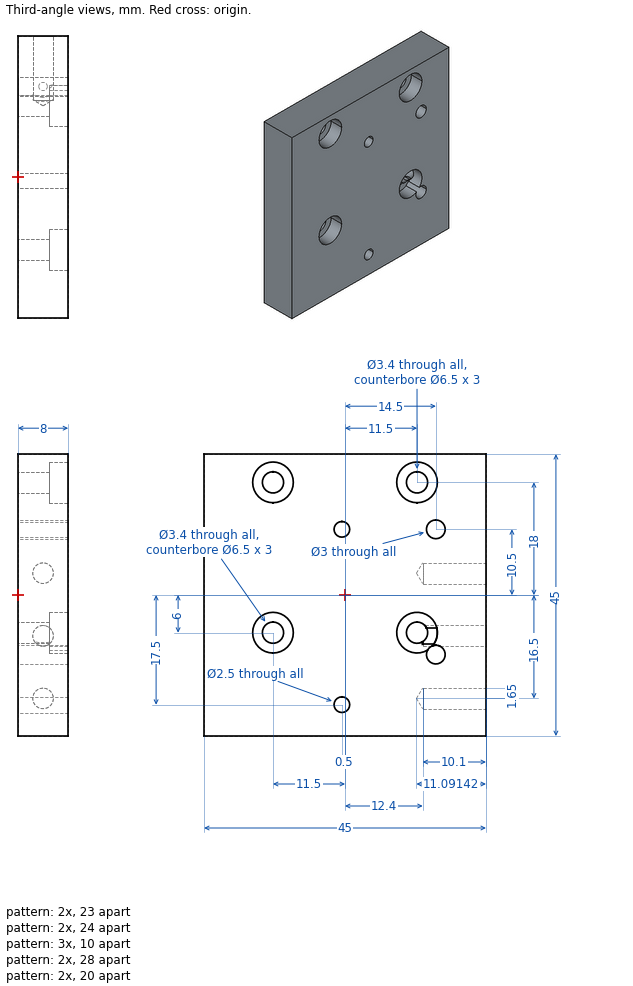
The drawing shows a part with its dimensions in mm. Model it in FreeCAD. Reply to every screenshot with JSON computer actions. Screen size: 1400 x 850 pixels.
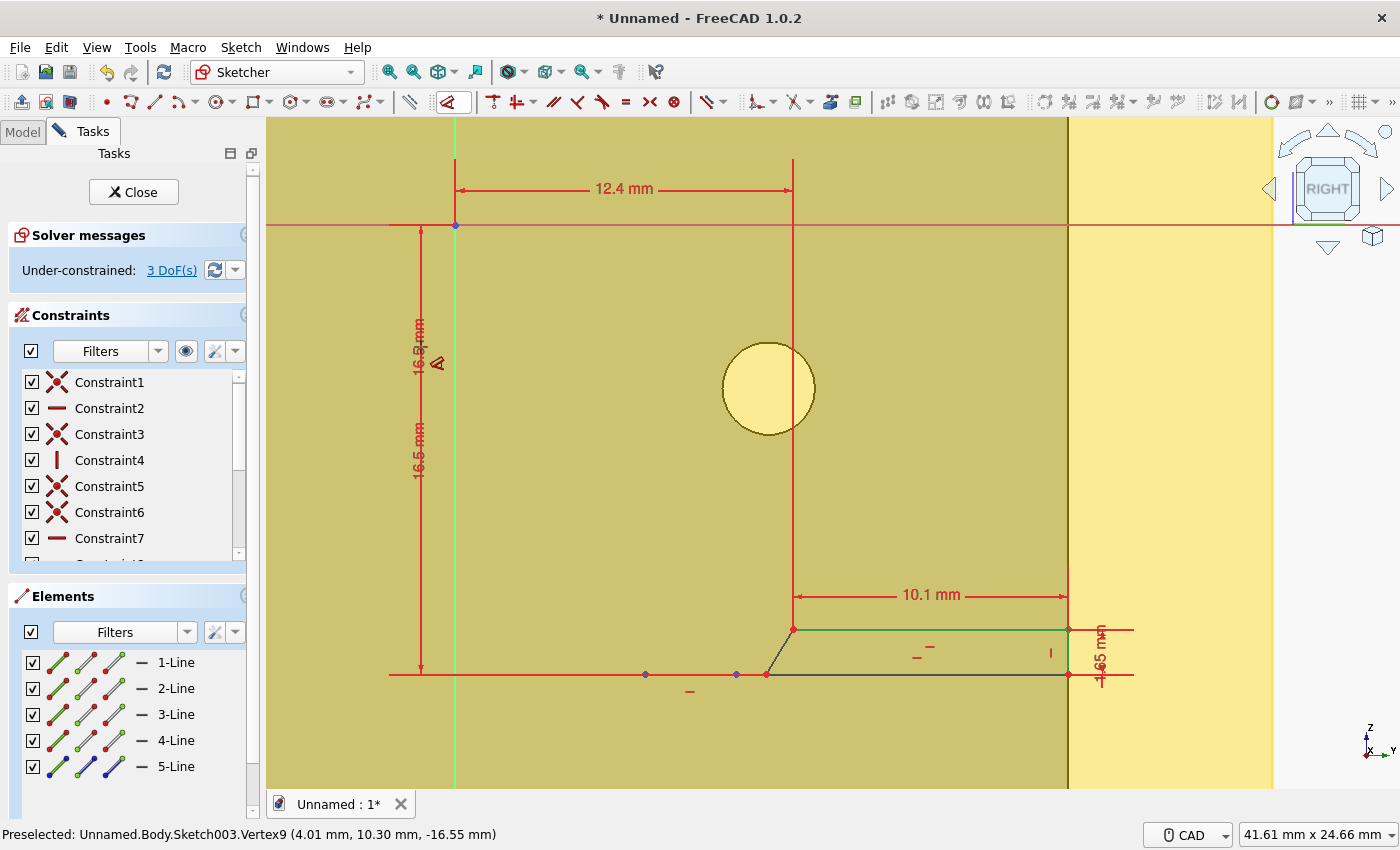
{"action": "left_click", "coordinate": [857, 675]}
{"action": "left_click", "coordinate": [917, 709]}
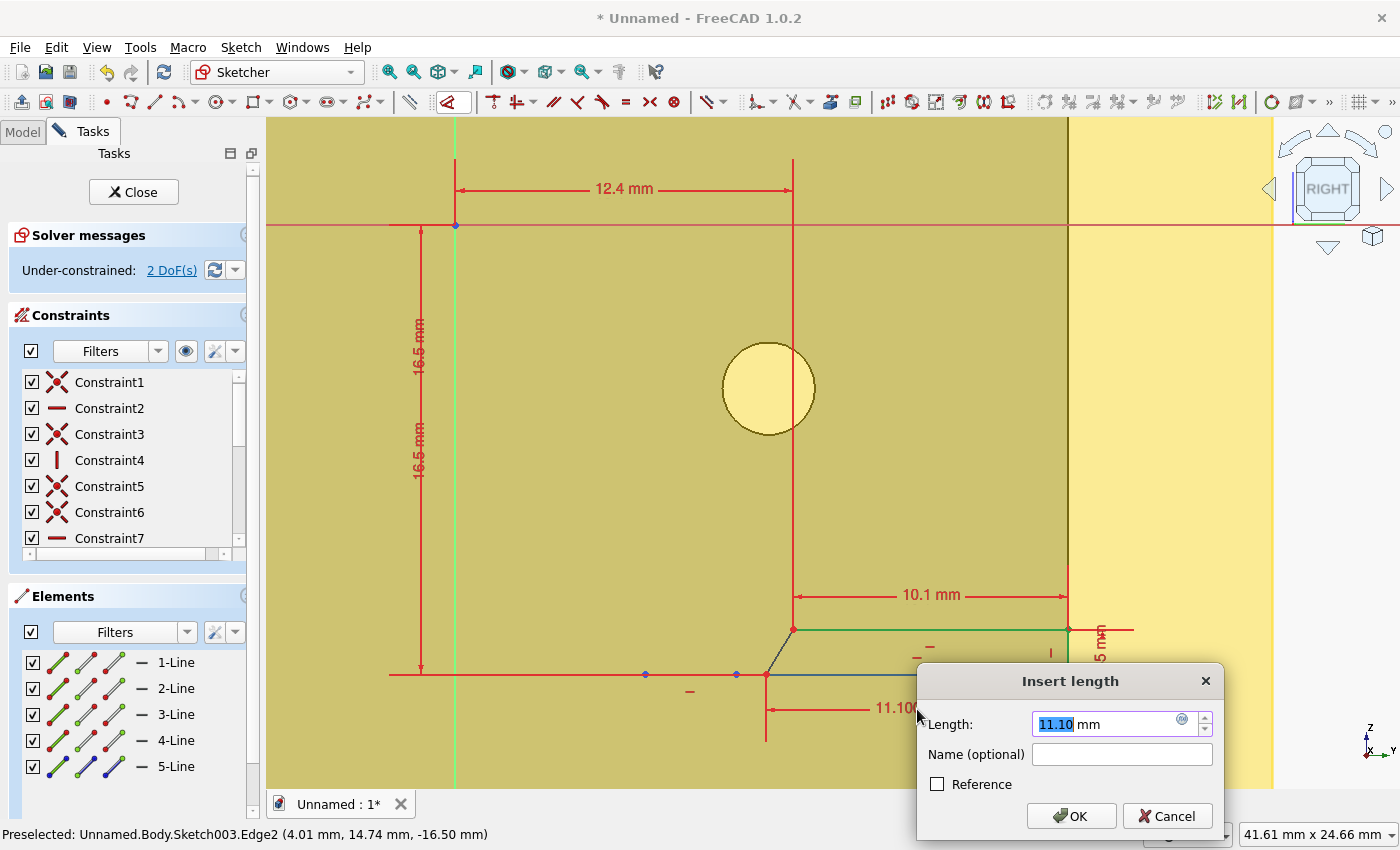
{"action": "type", "text": "11.09142"}
{"action": "key", "text": "Return"}
{"action": "key", "text": "Escape"}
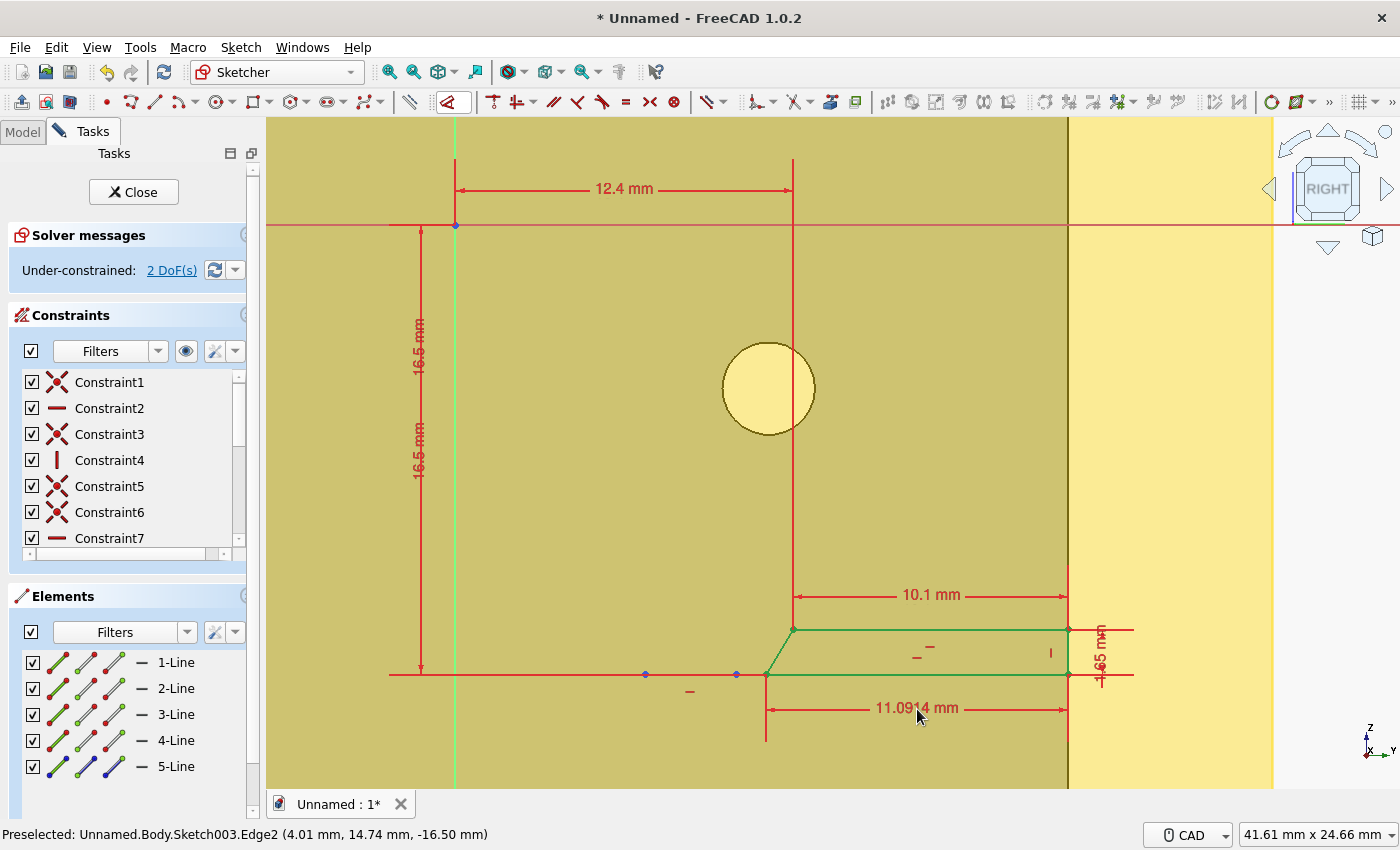
{"action": "left_click", "coordinate": [134, 192]}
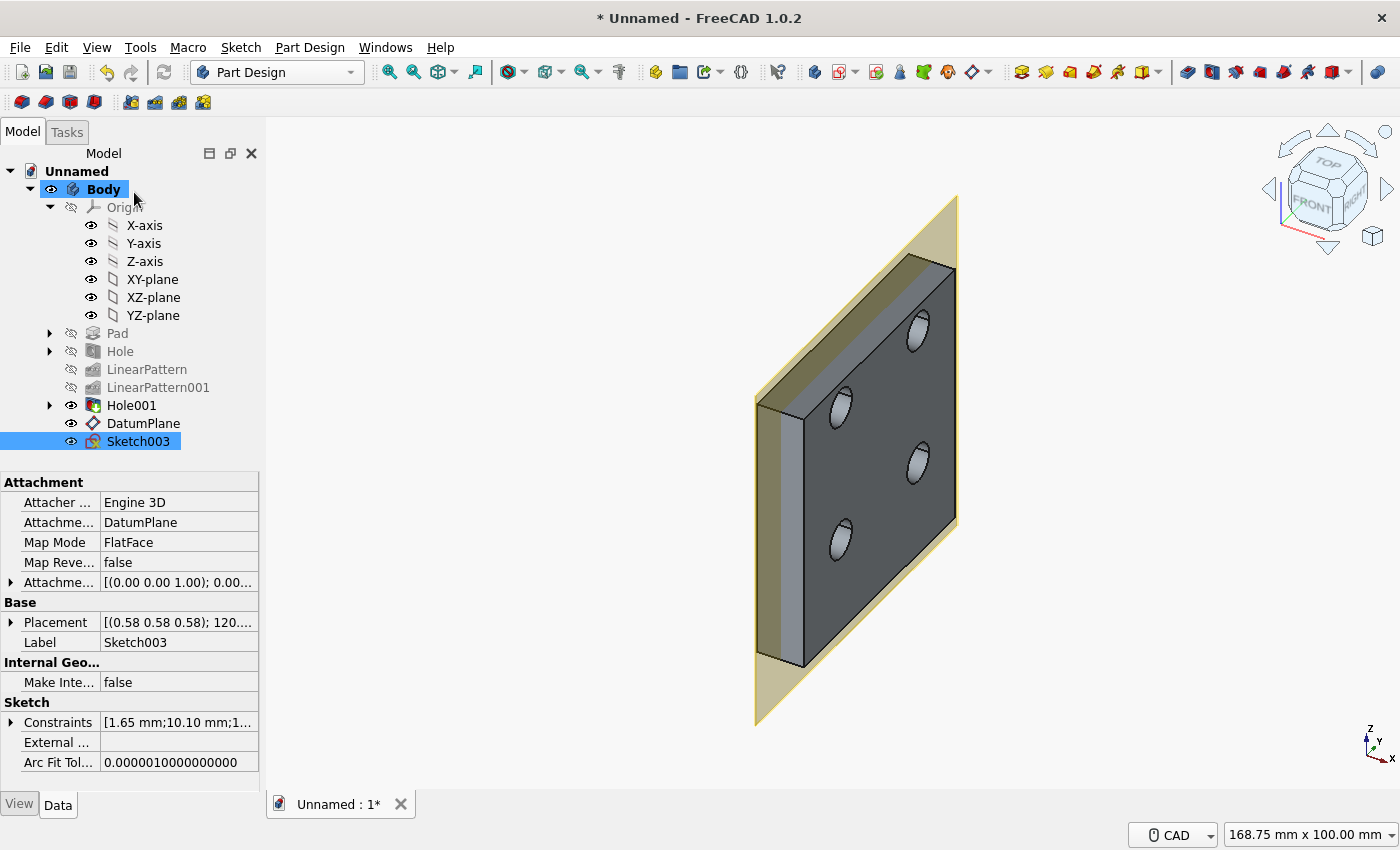
{"action": "left_click", "coordinate": [1236, 72]}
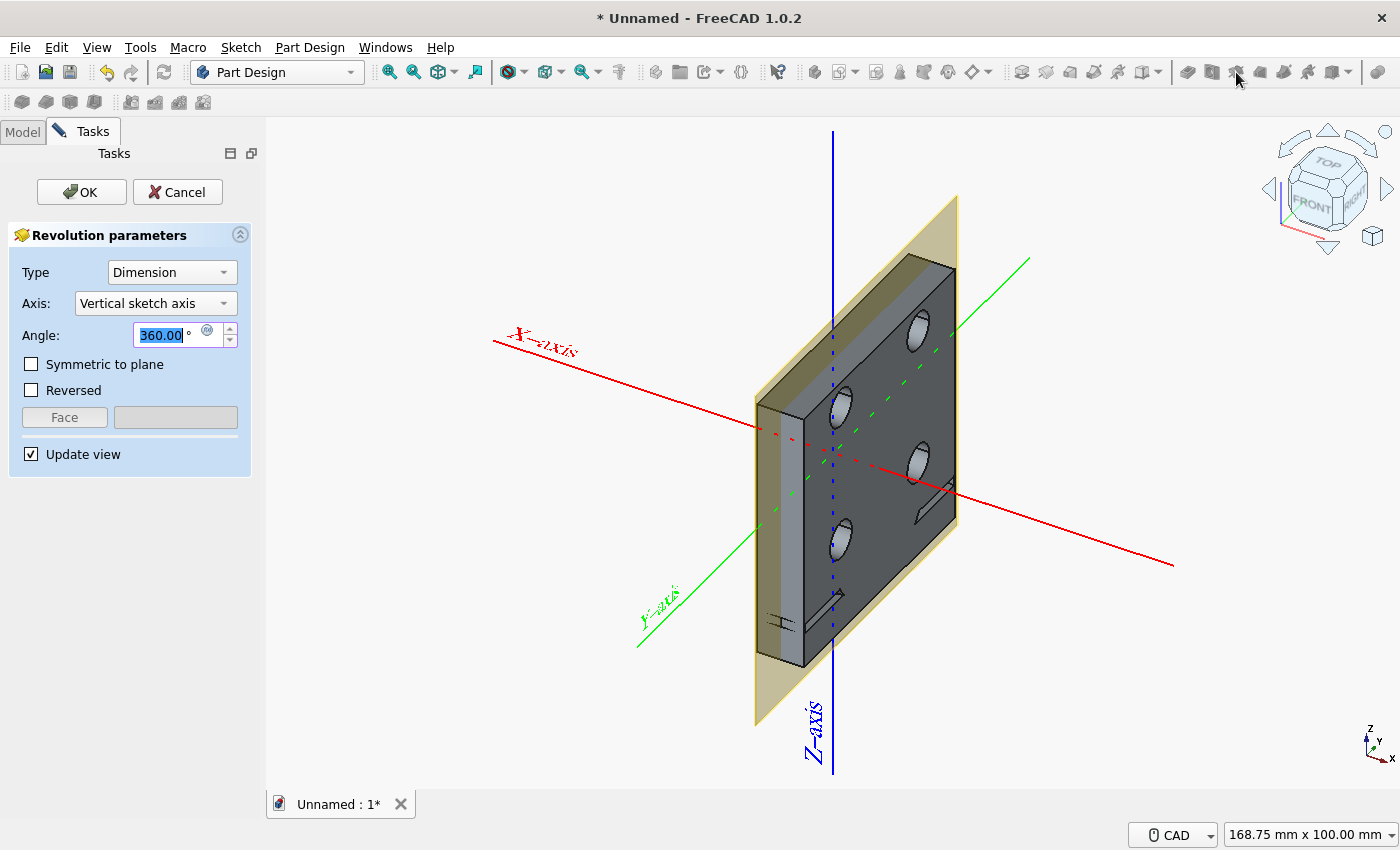
{"action": "left_click", "coordinate": [156, 304]}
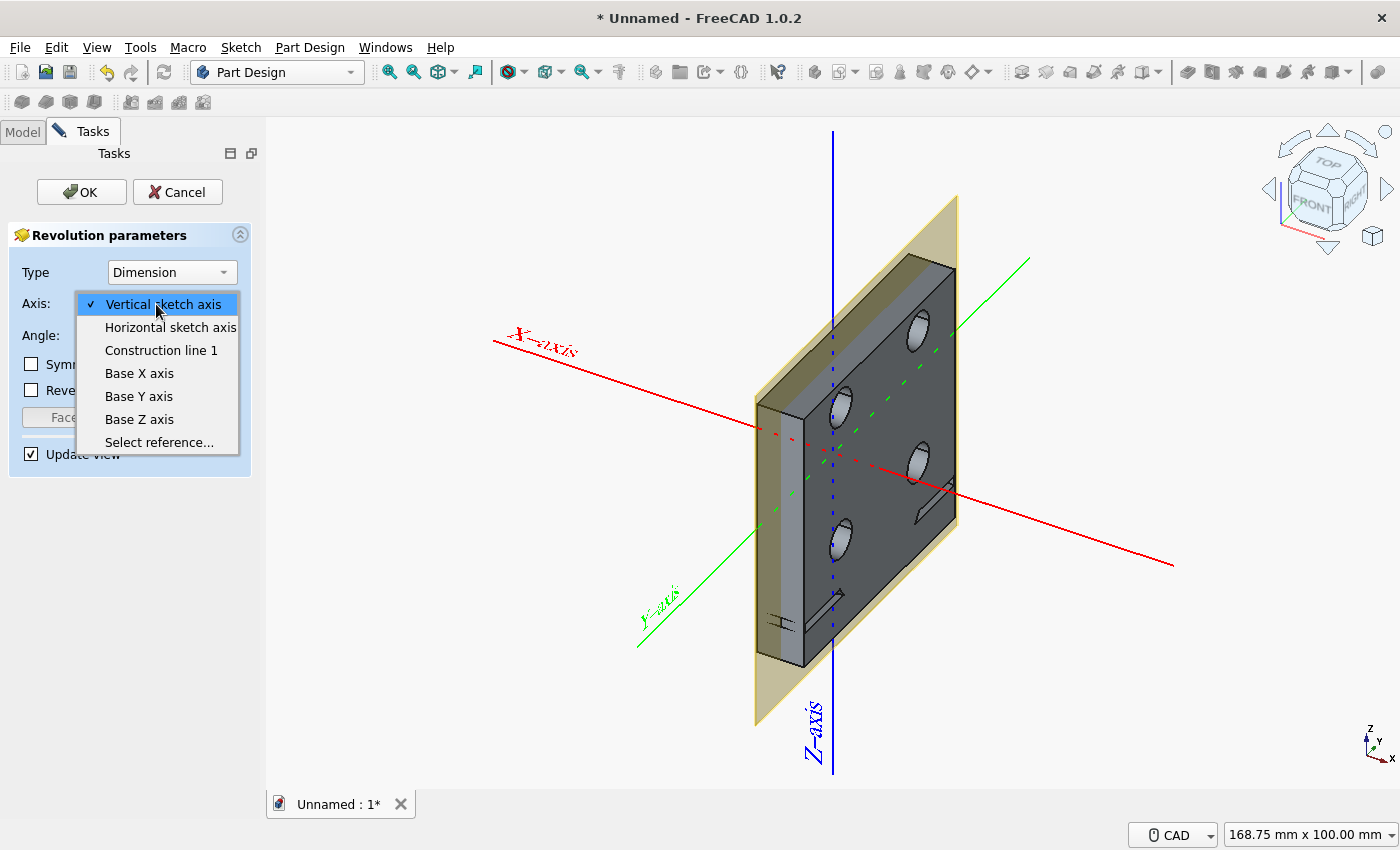
{"action": "left_click", "coordinate": [156, 350]}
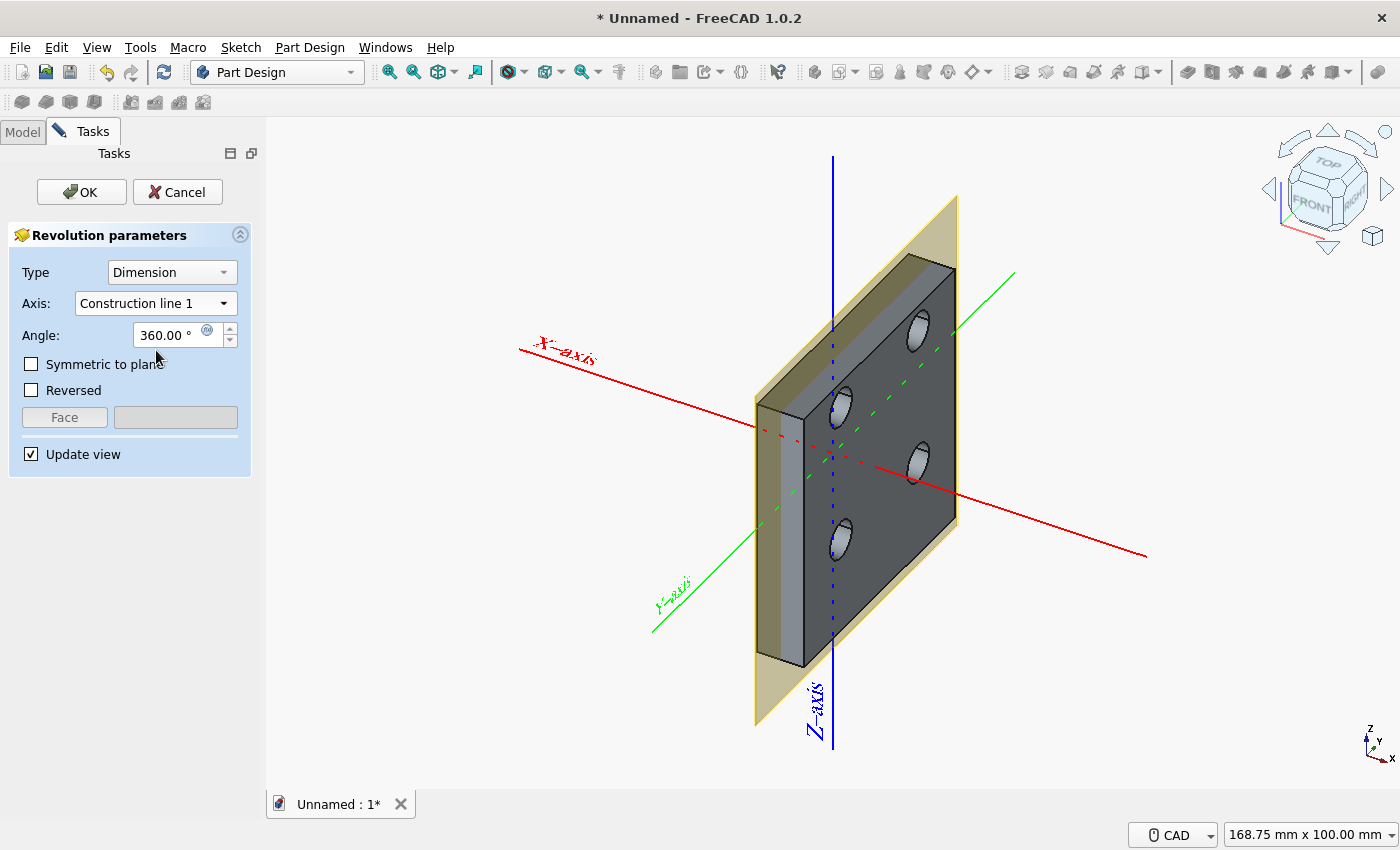
{"action": "left_click", "coordinate": [82, 192]}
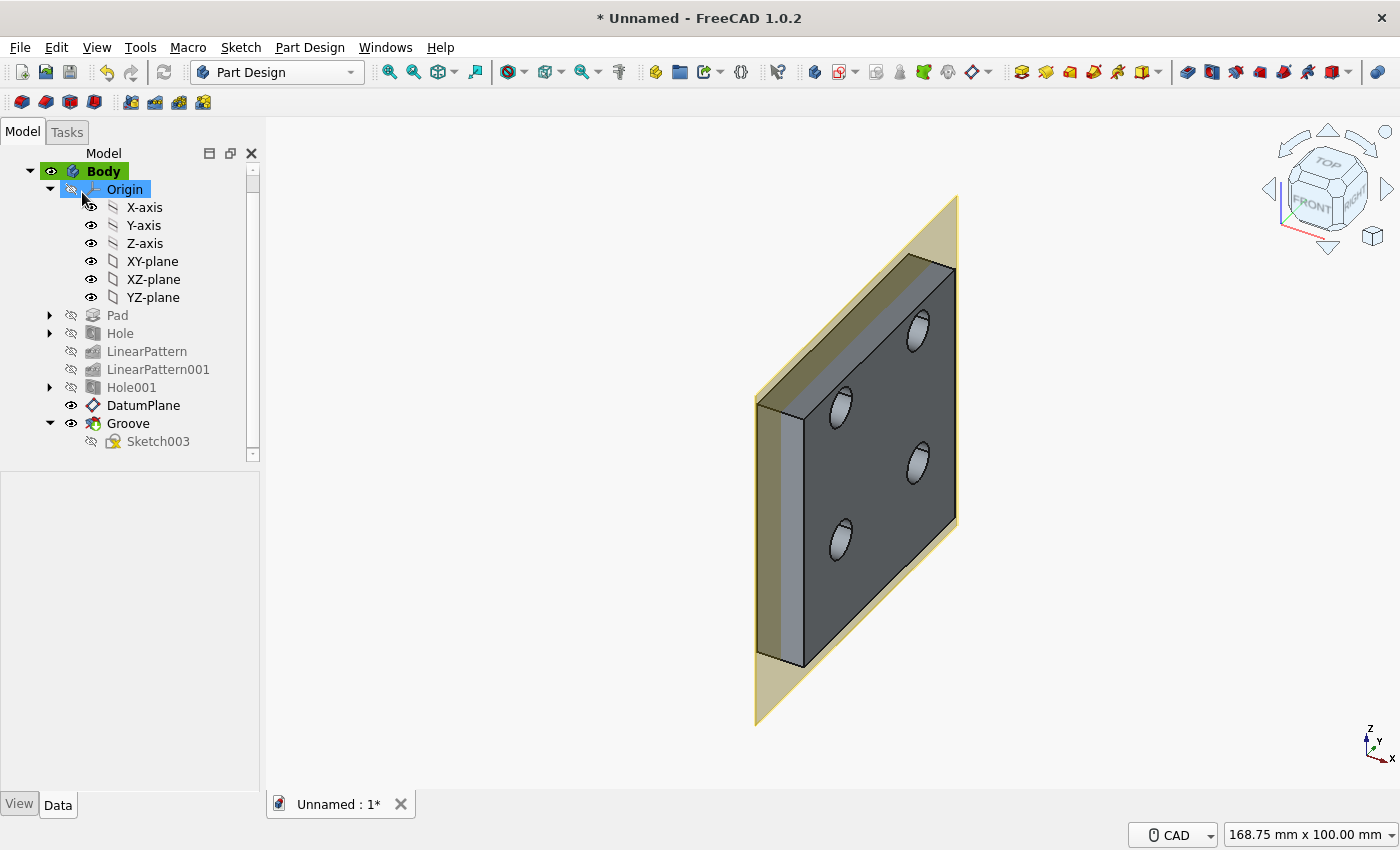
{"action": "left_click", "coordinate": [116, 405]}
{"action": "key", "text": "space"}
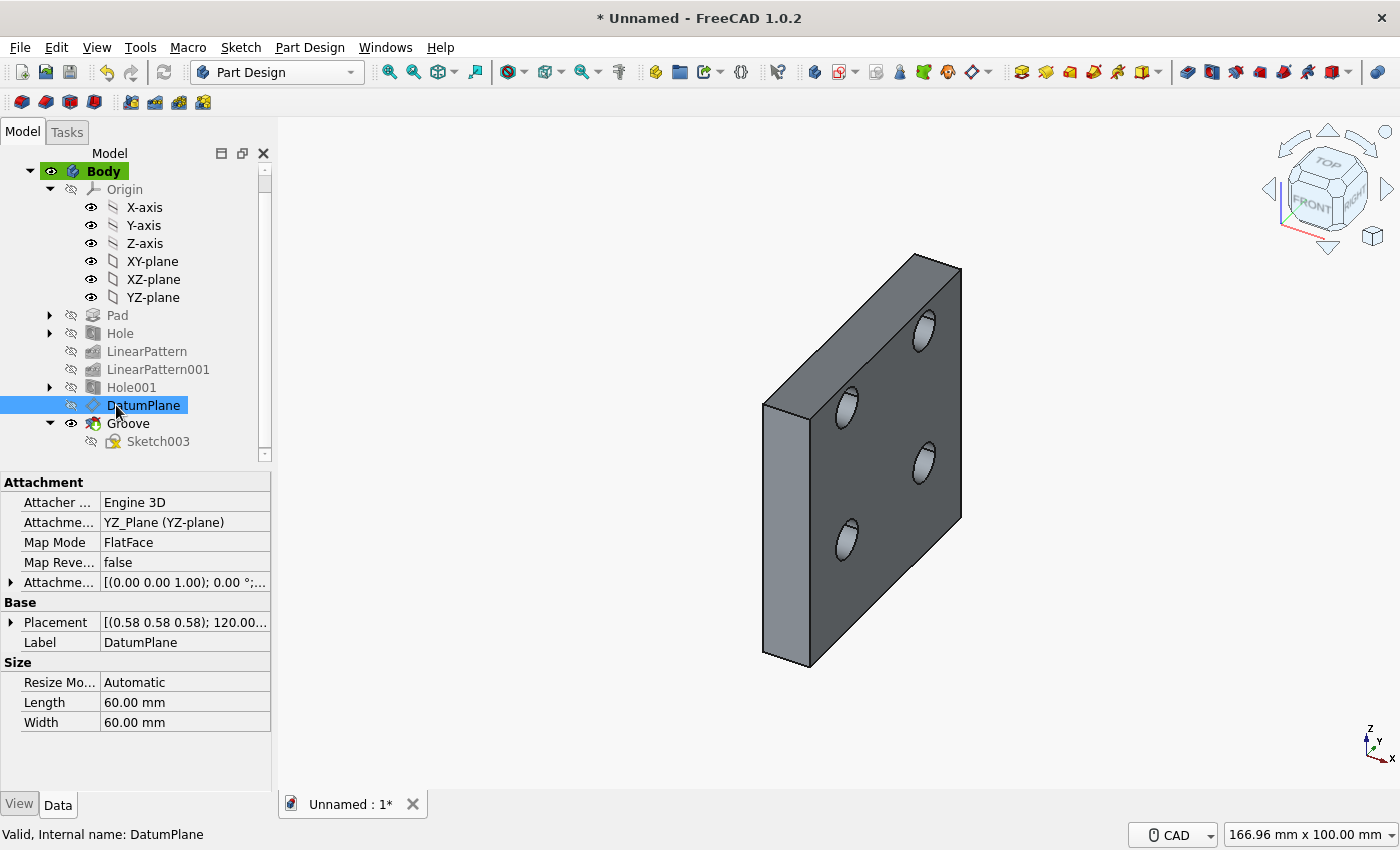
{"action": "left_click", "coordinate": [116, 423]}